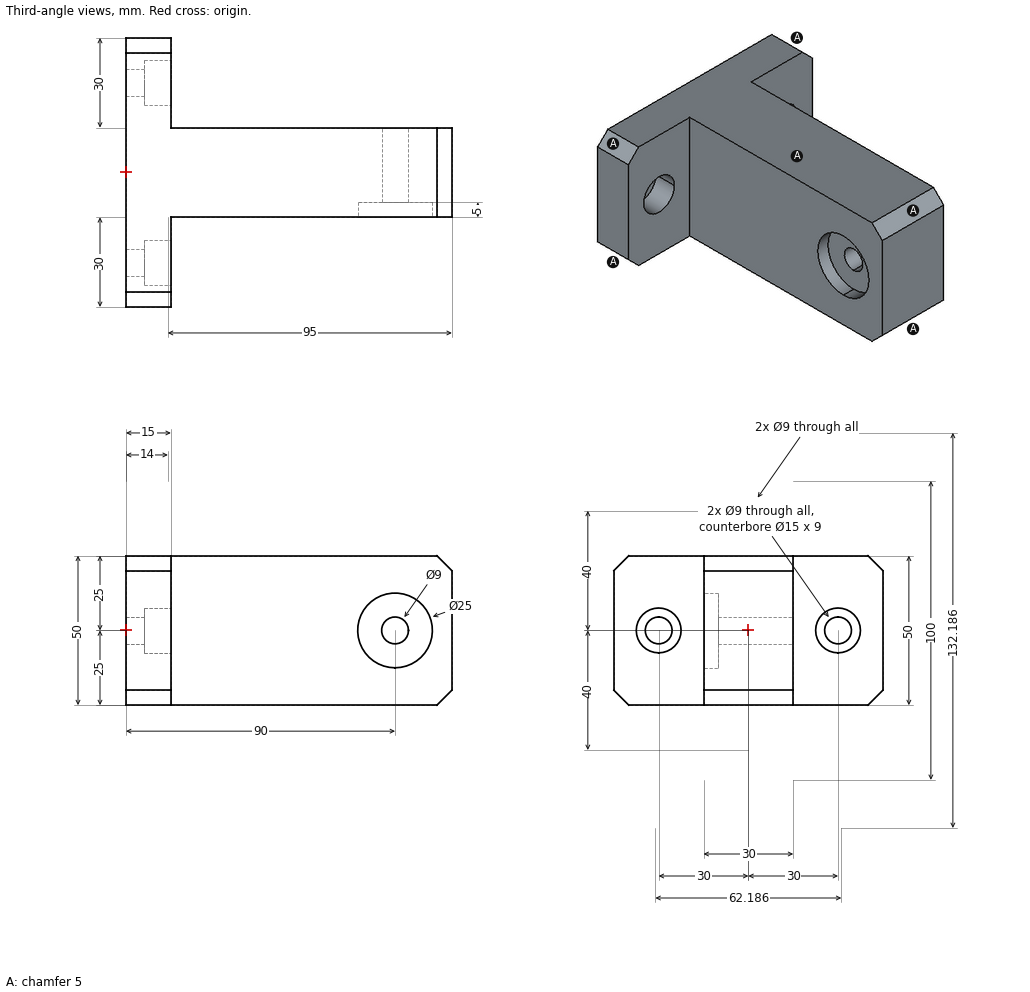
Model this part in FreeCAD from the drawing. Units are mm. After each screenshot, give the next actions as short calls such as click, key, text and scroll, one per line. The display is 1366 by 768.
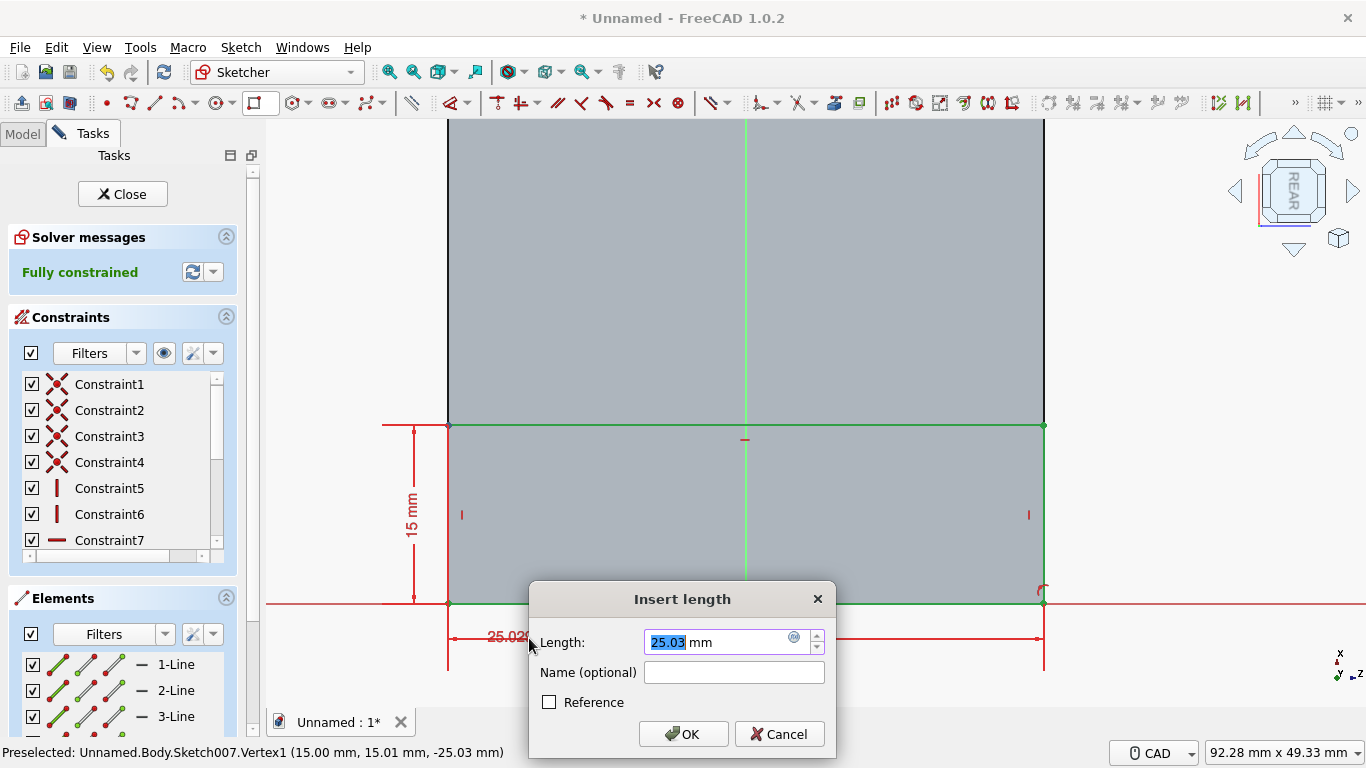
text(25)
key(Return)
key(Escape)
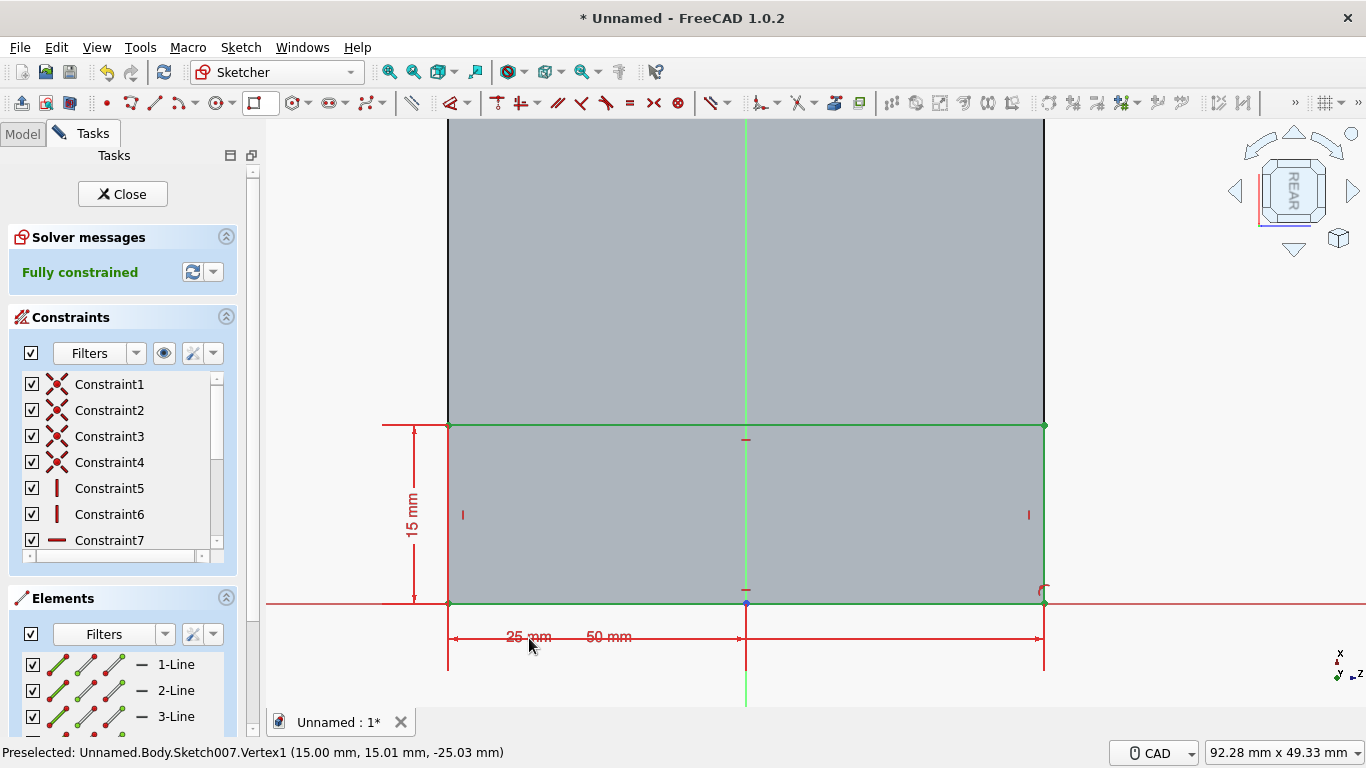
click(123, 194)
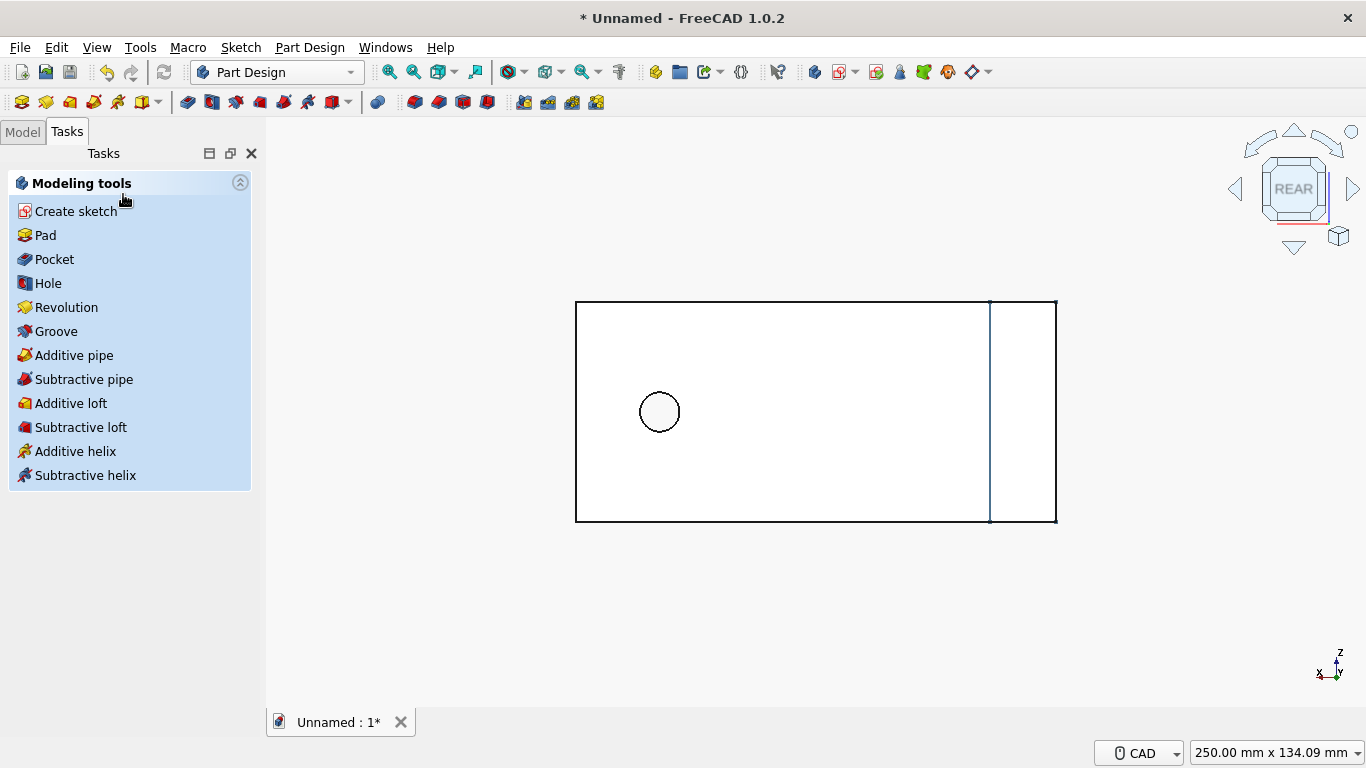
click(22, 102)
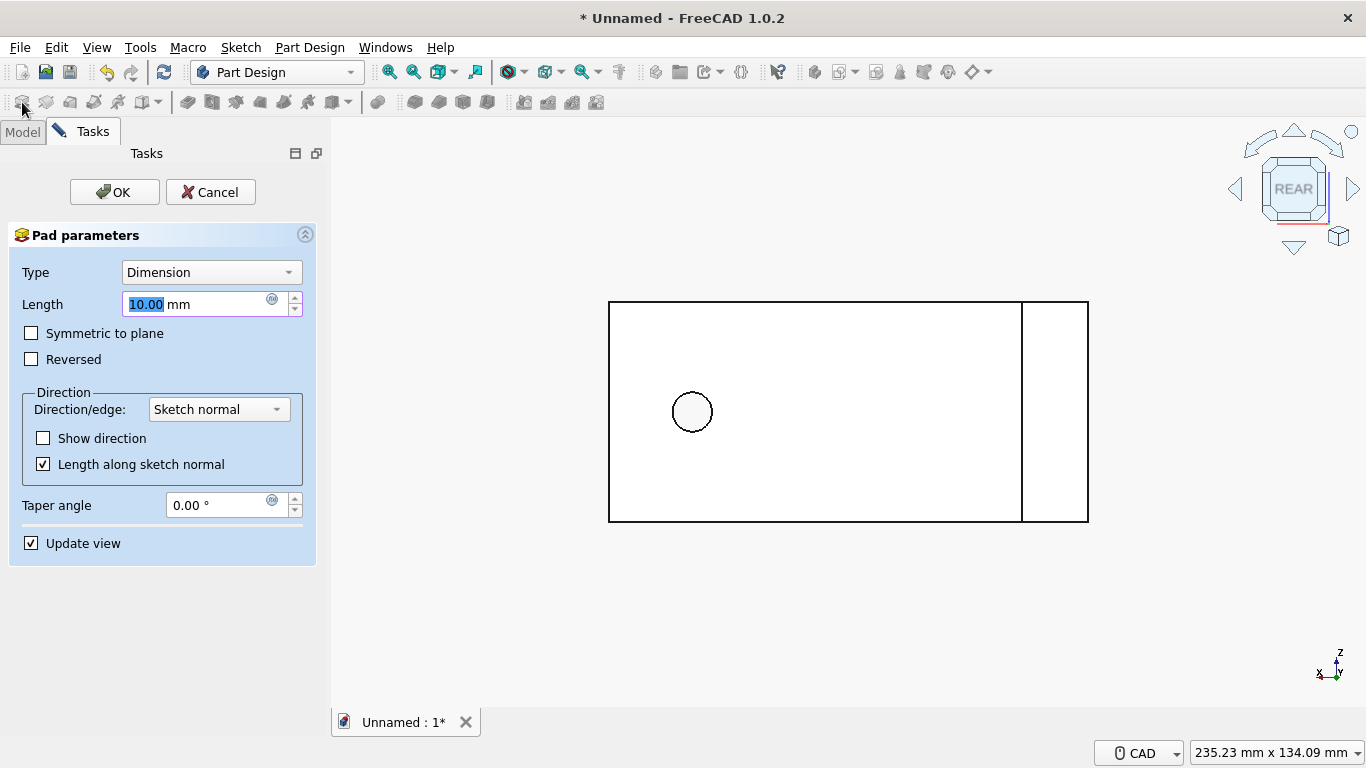
text(30)
key(Tab)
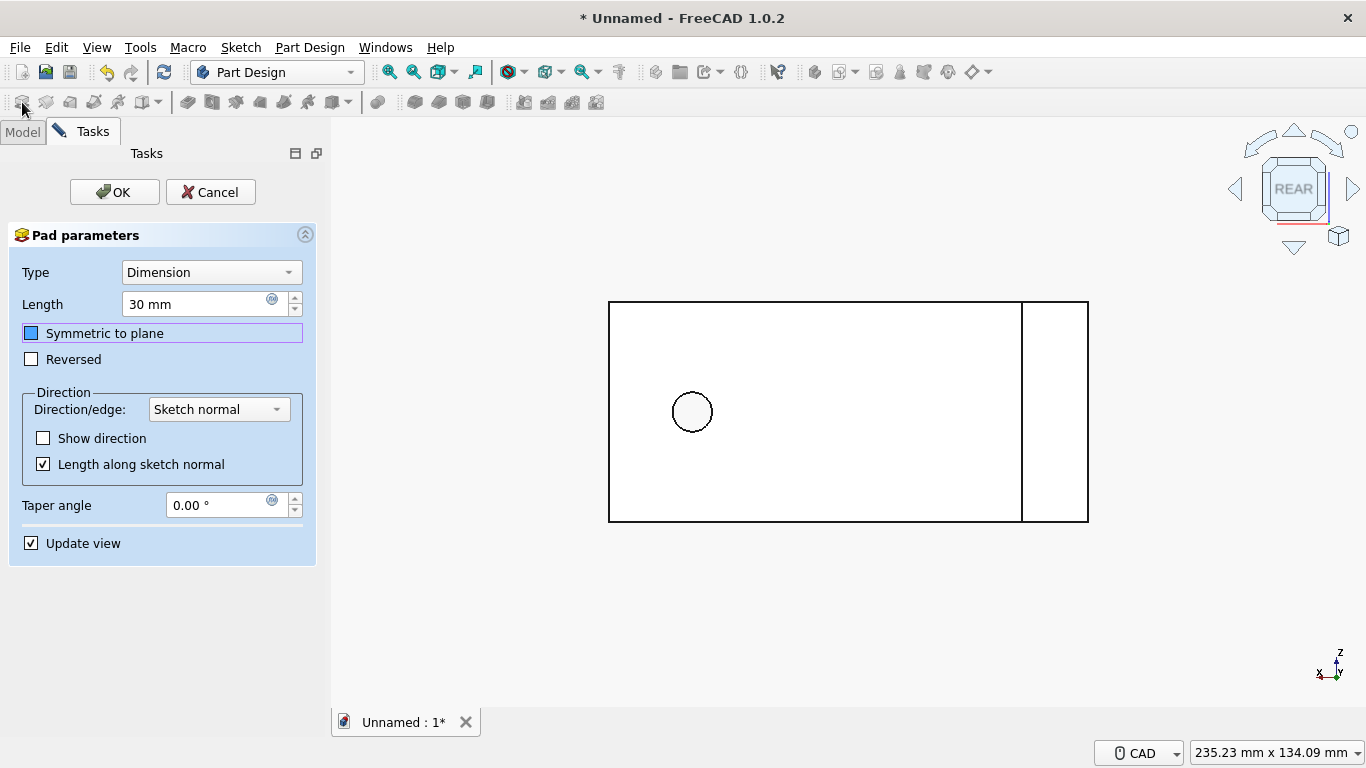
click(115, 192)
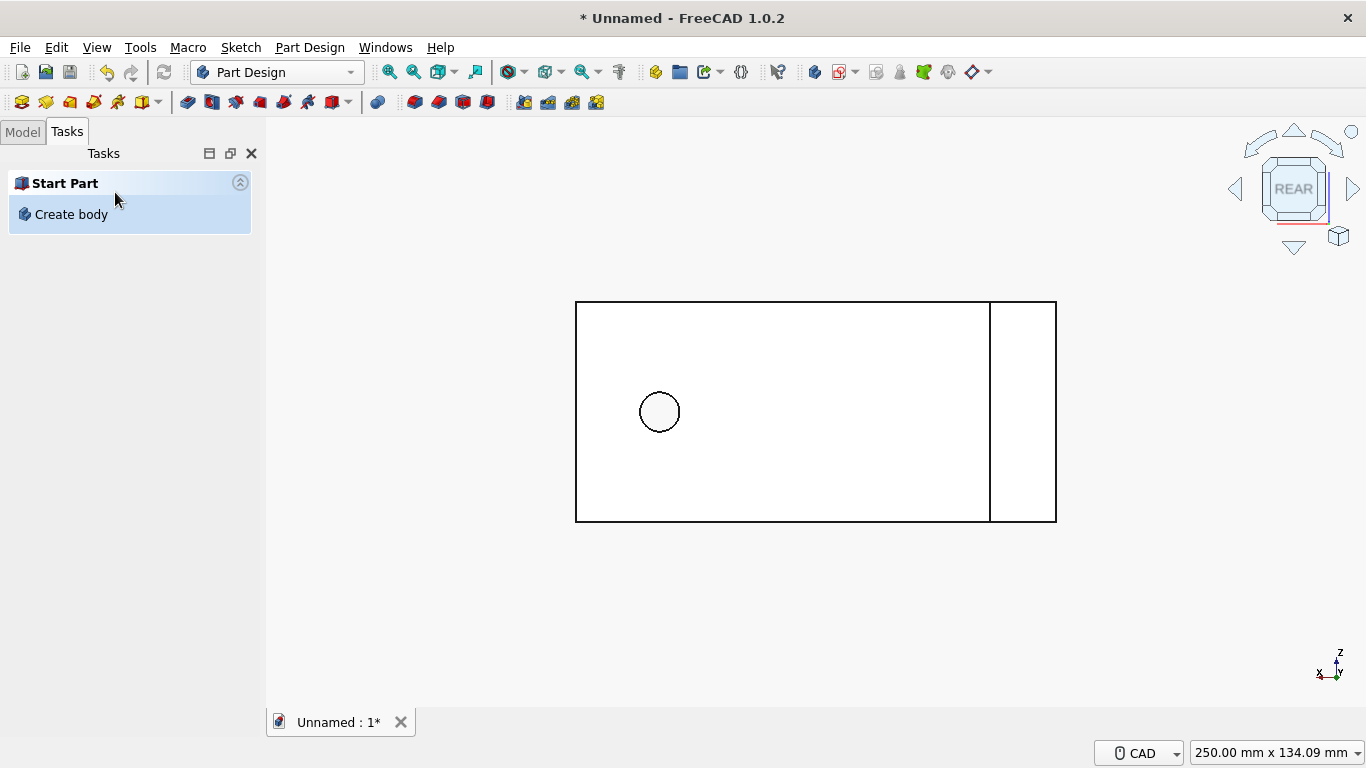
click(390, 72)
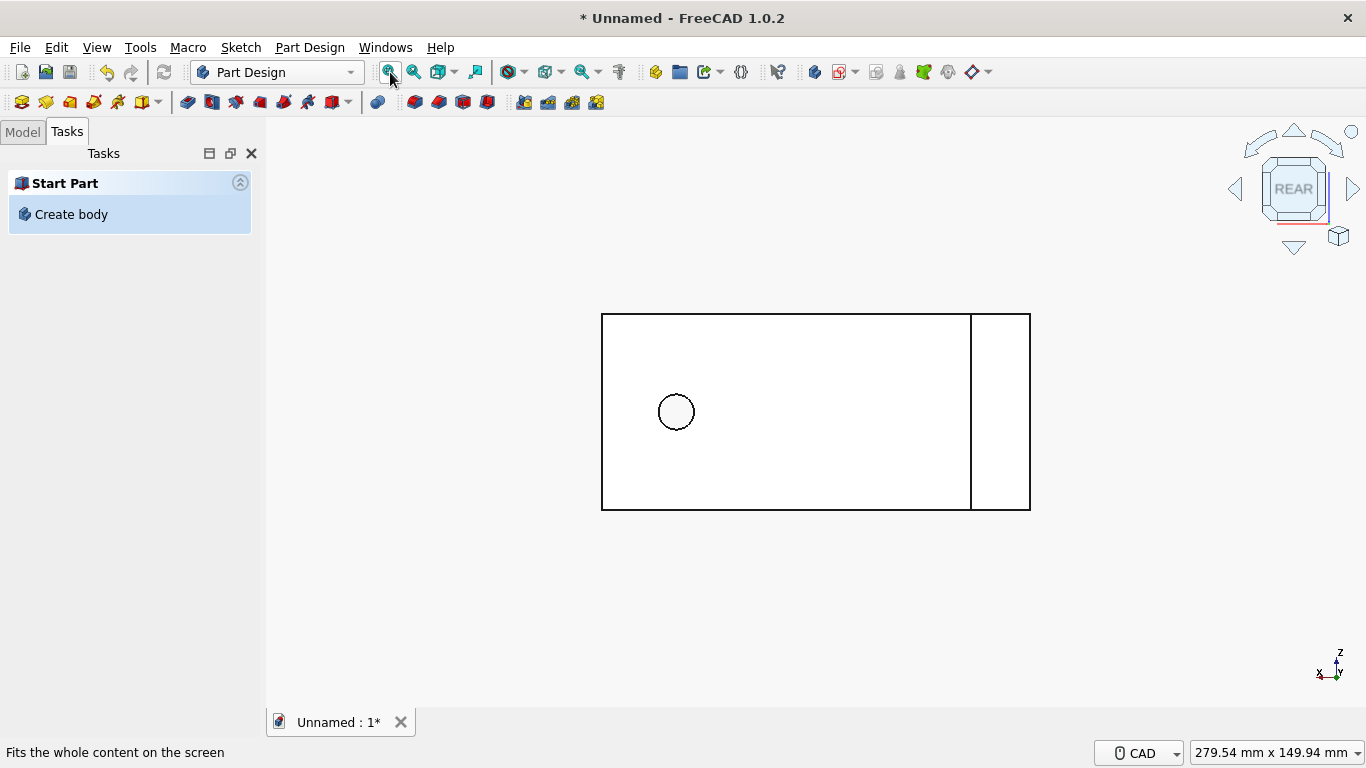
key(0)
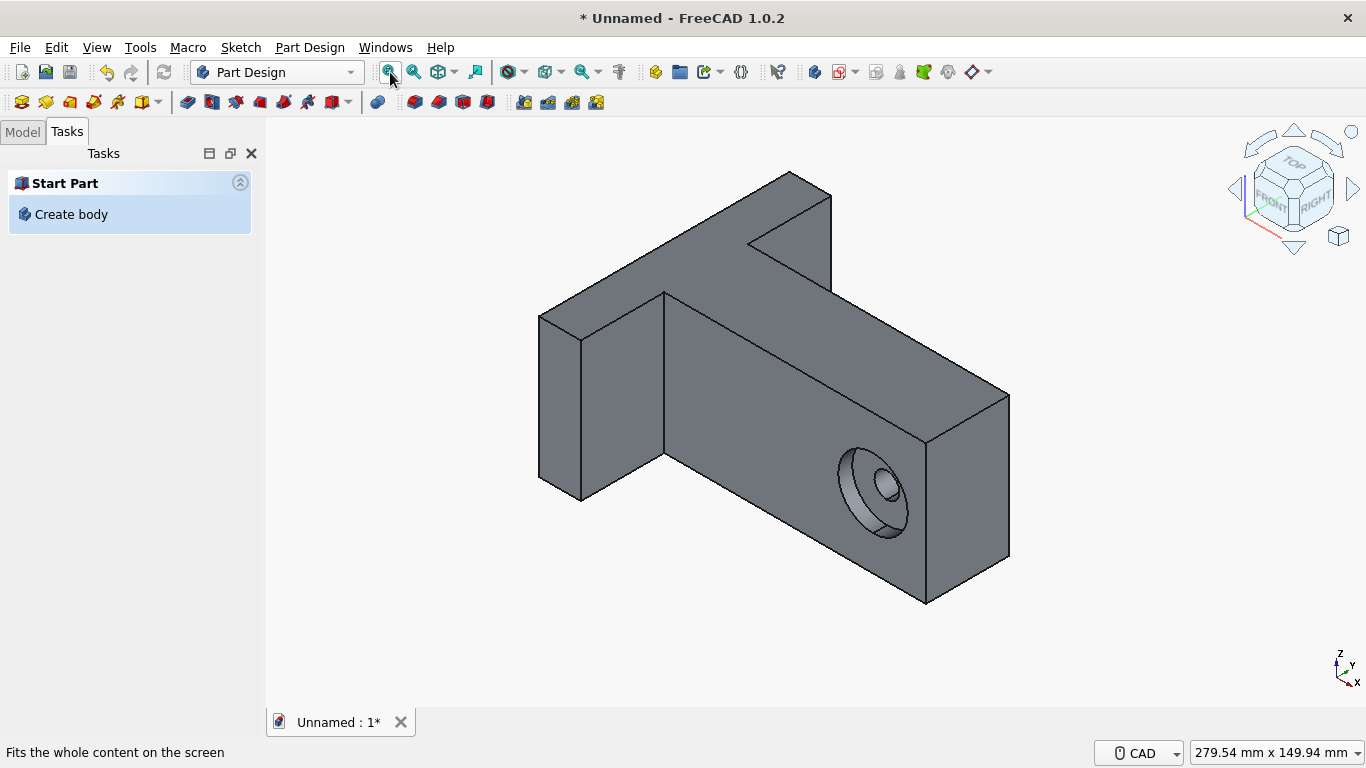
click(623, 396)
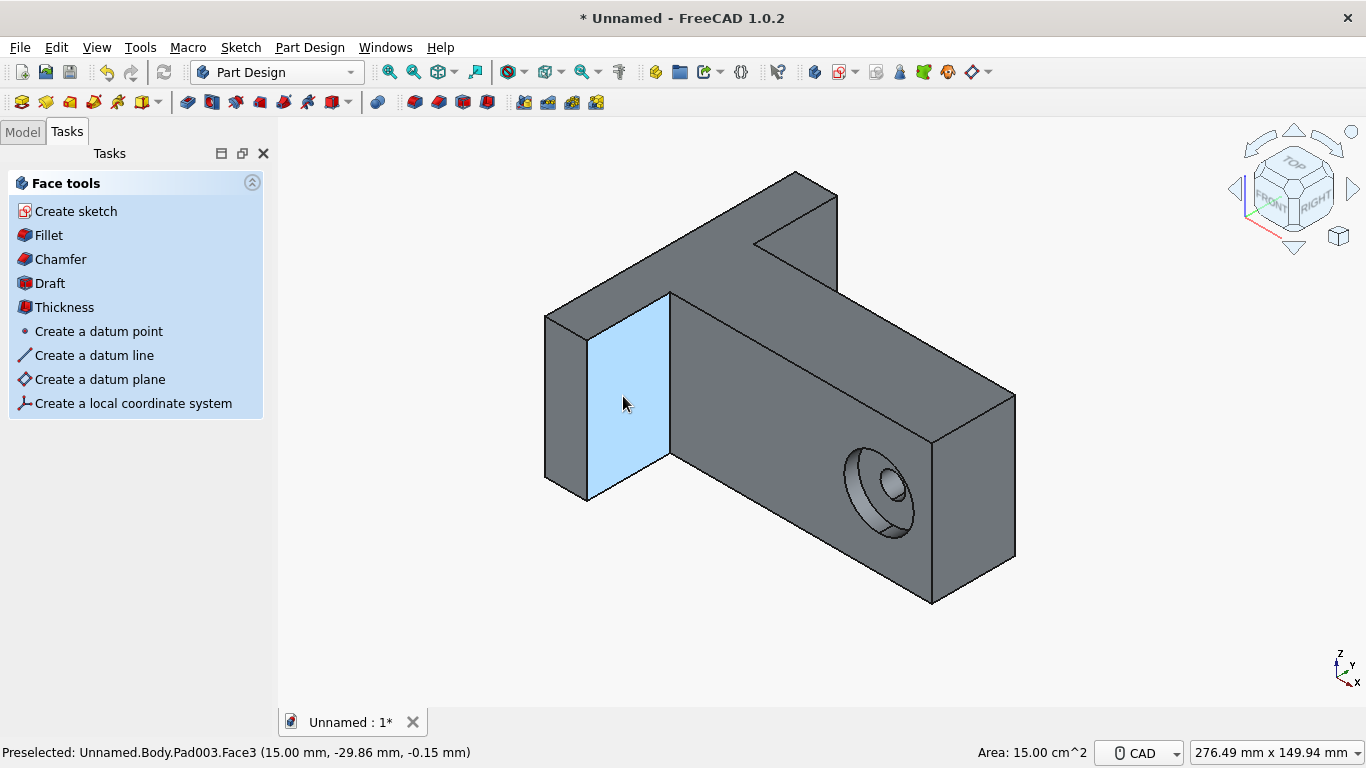
click(840, 72)